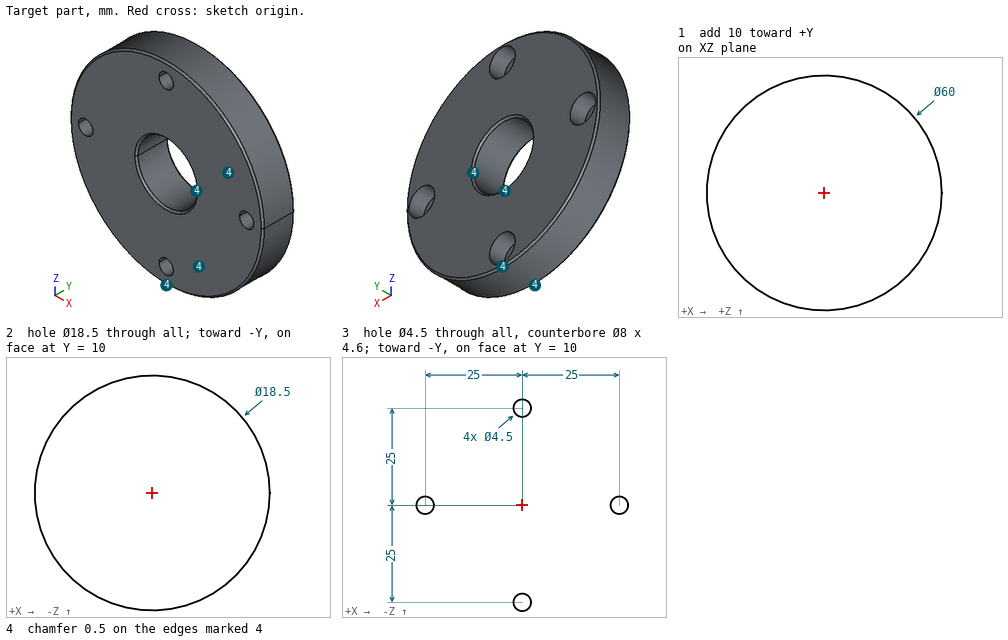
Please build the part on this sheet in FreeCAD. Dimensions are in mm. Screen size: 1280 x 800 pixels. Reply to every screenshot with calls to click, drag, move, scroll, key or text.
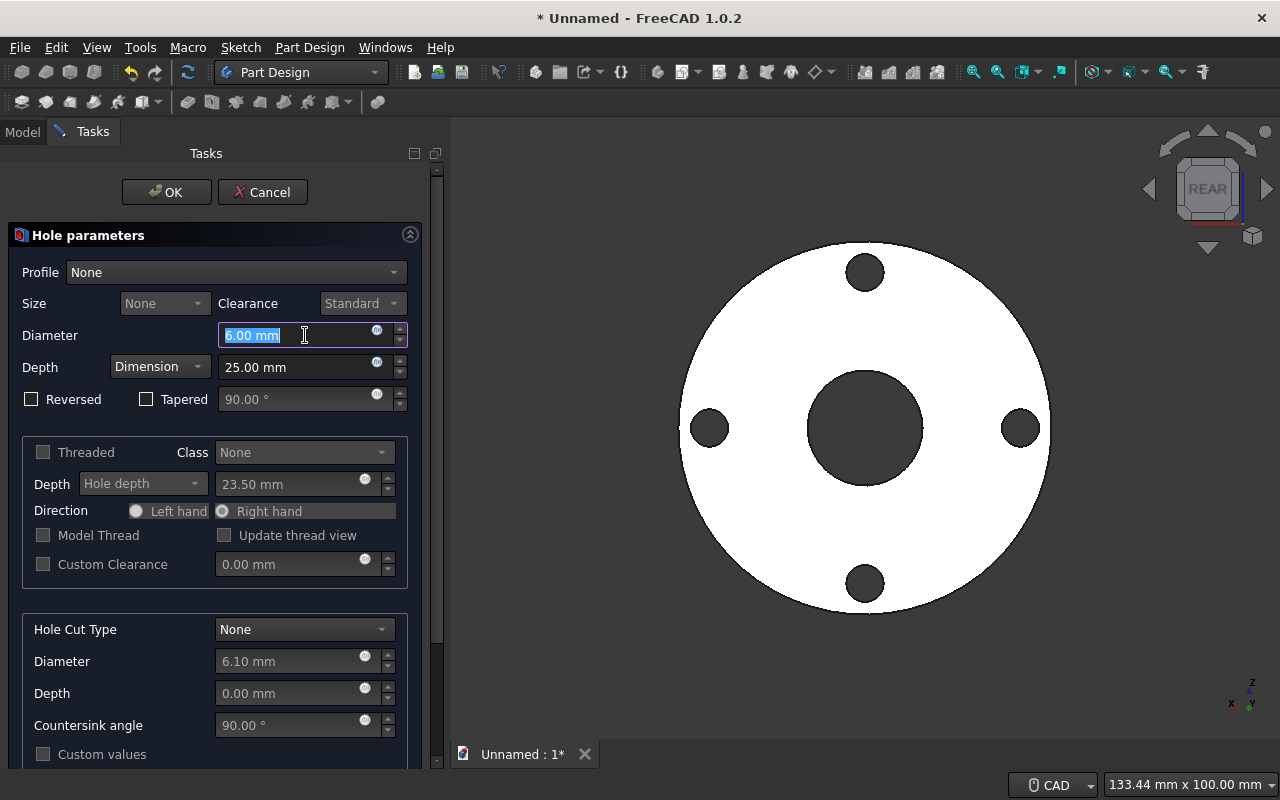
text(4.5)
key(Tab)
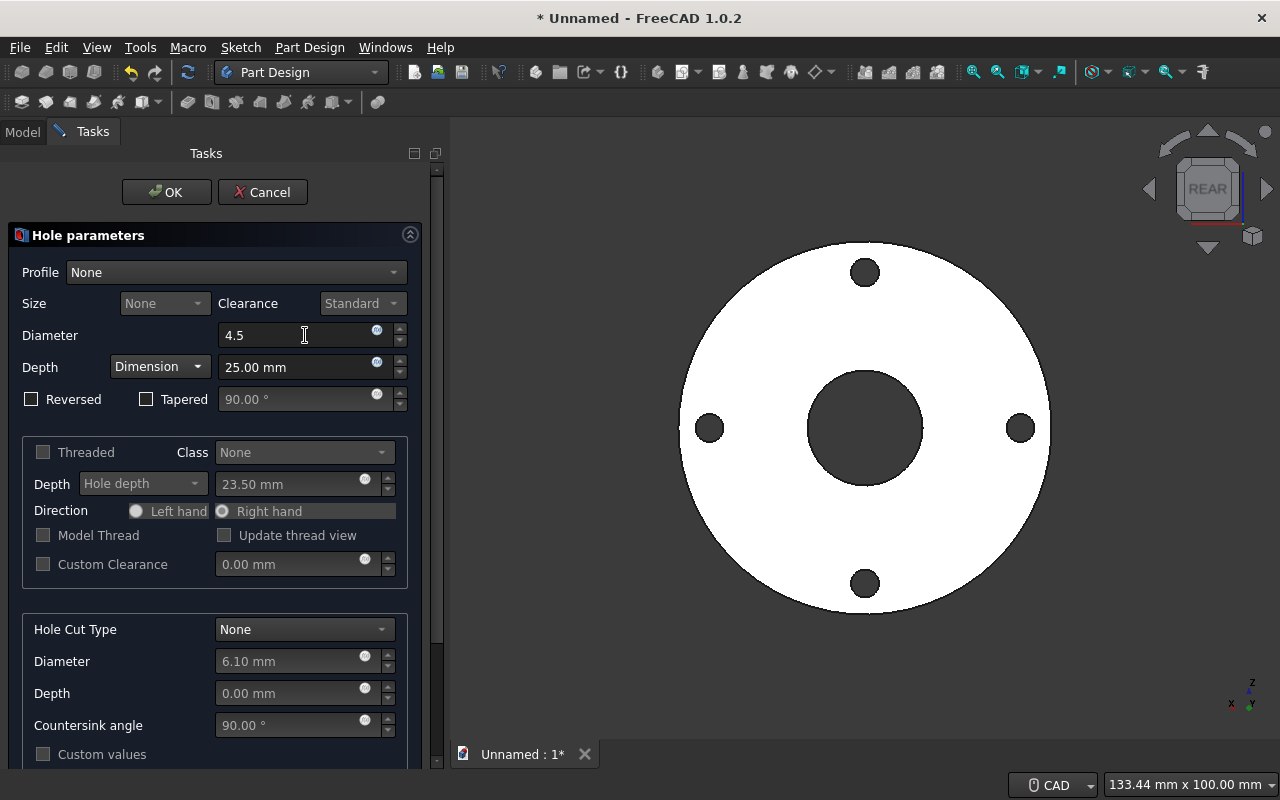
click(161, 366)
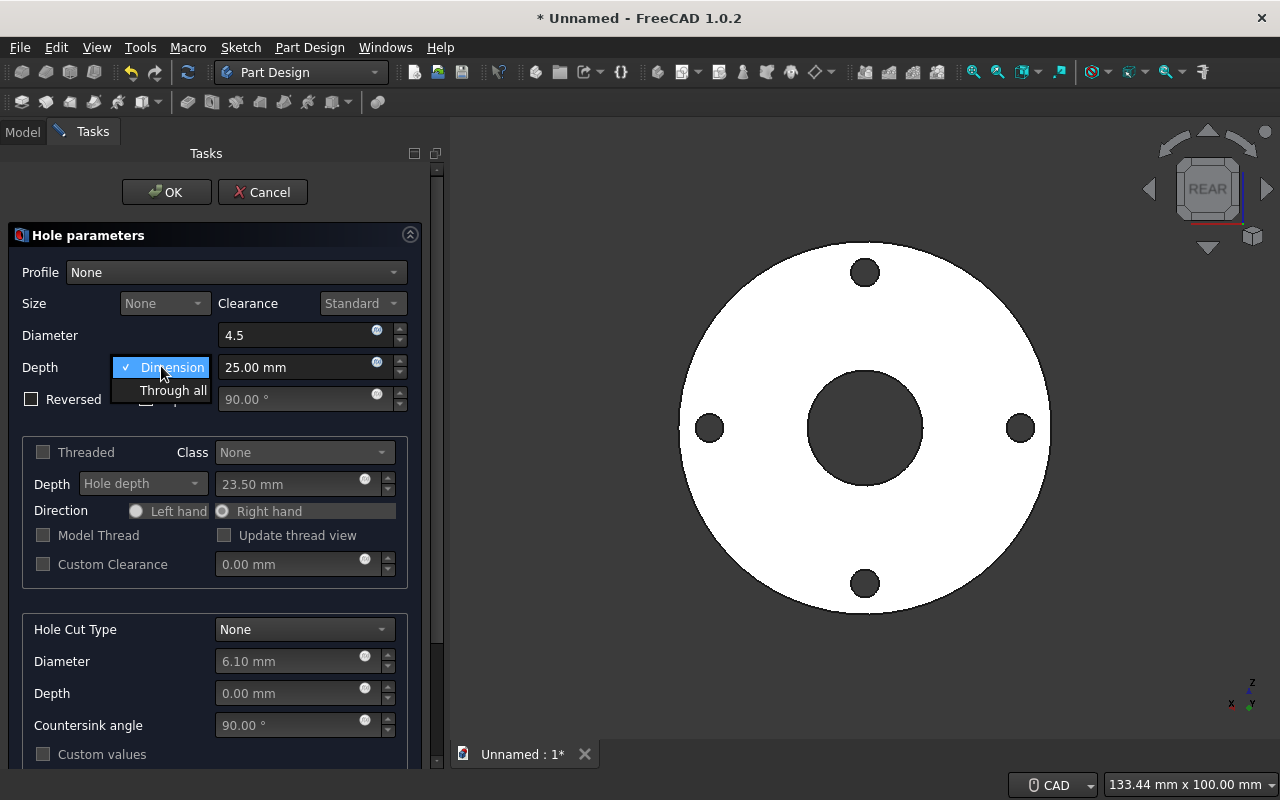
click(160, 390)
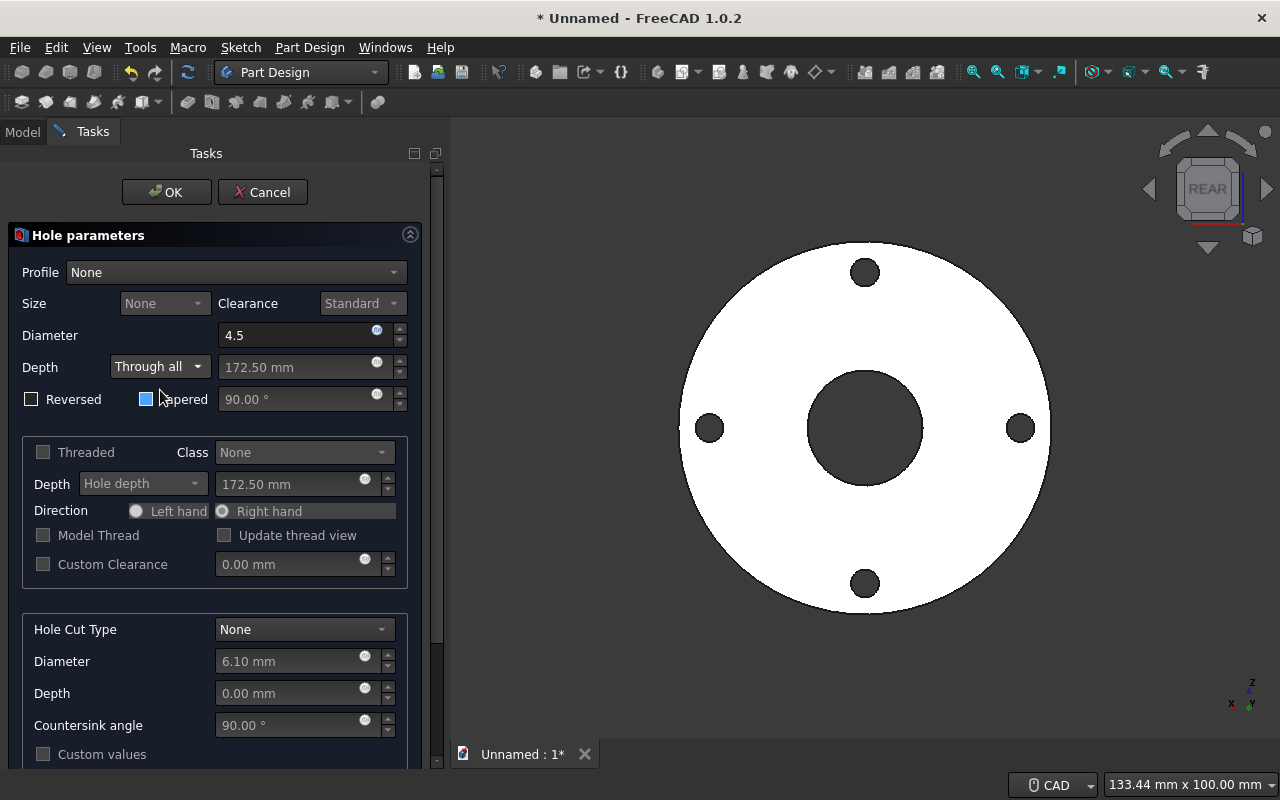
click(306, 630)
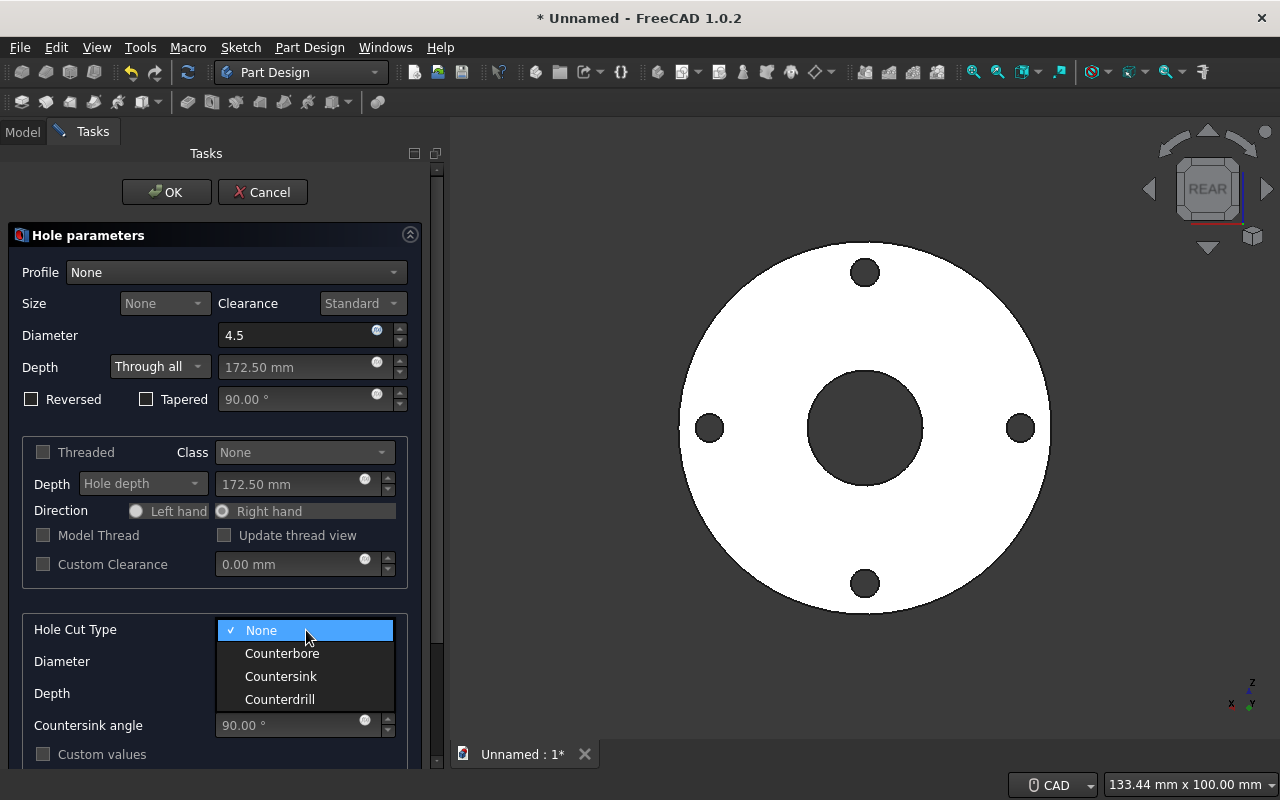
click(304, 654)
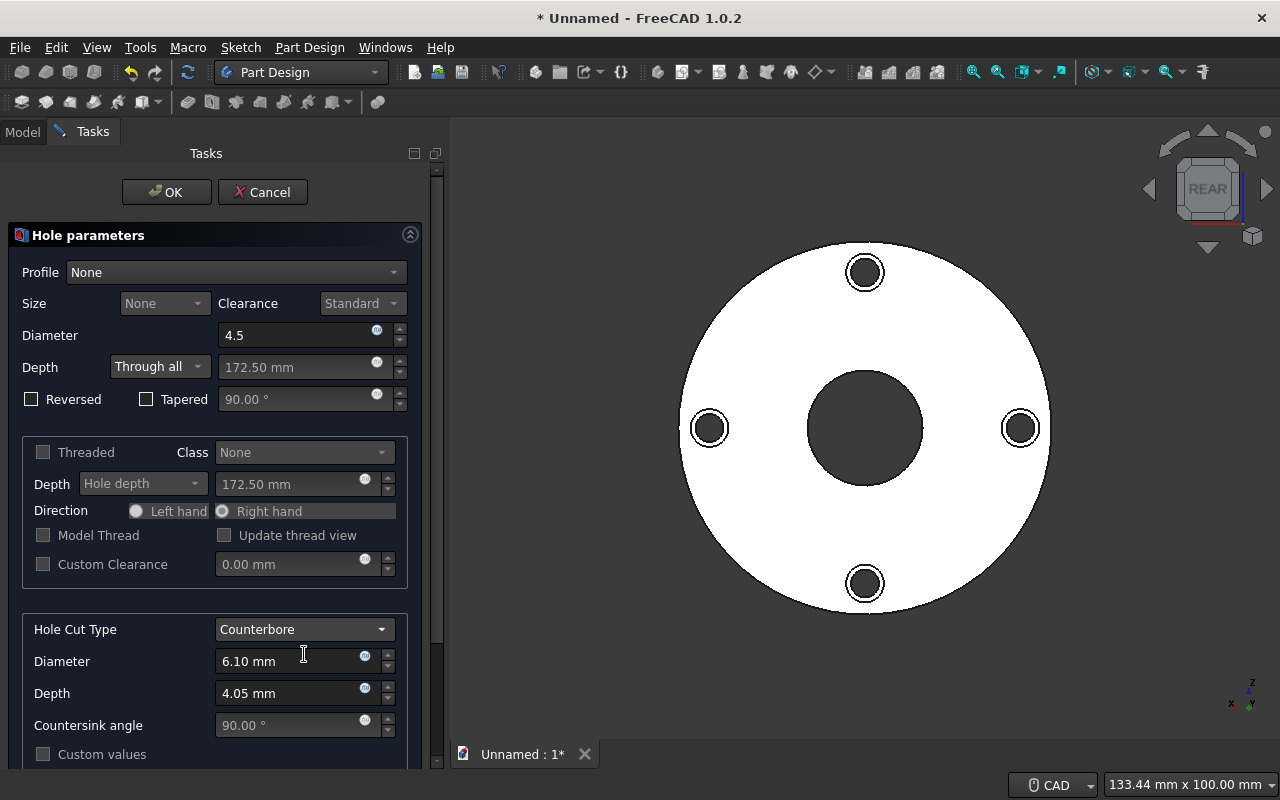
triple_click(298, 661)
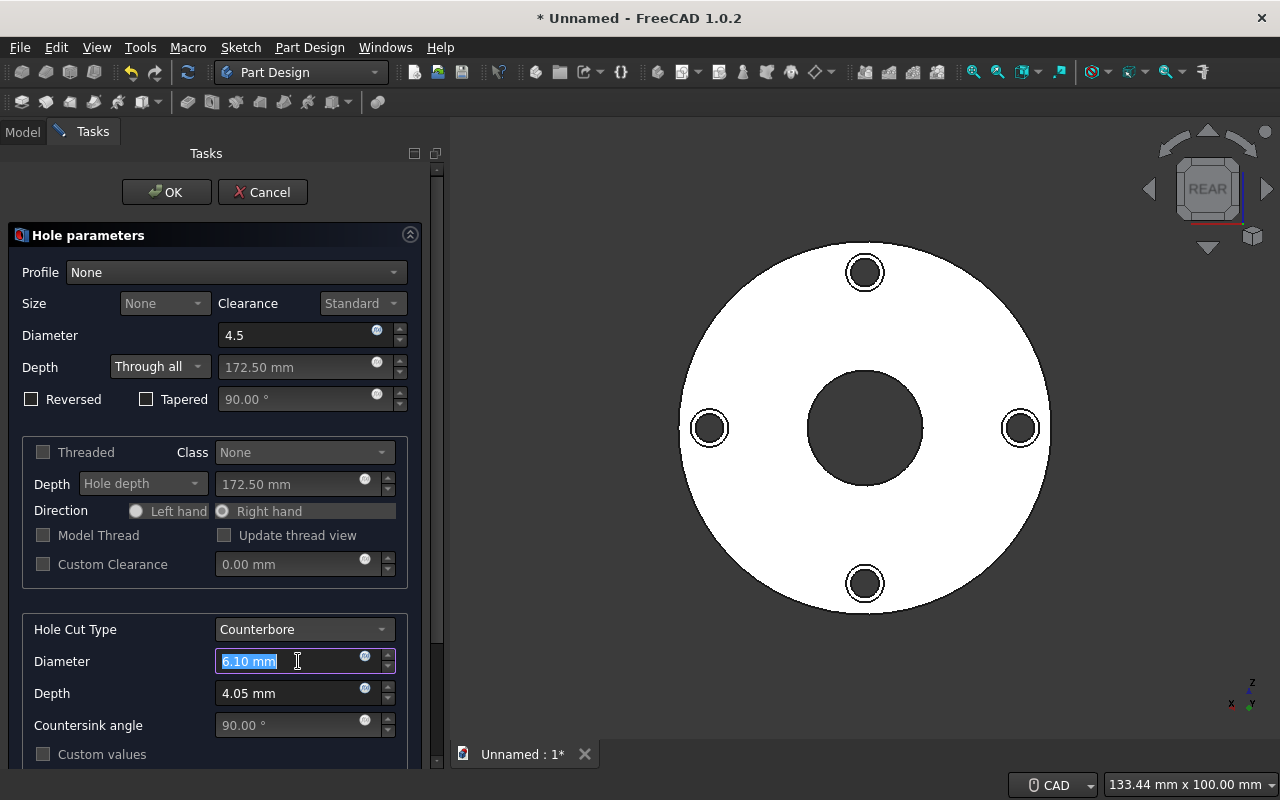
text(8)
key(Tab)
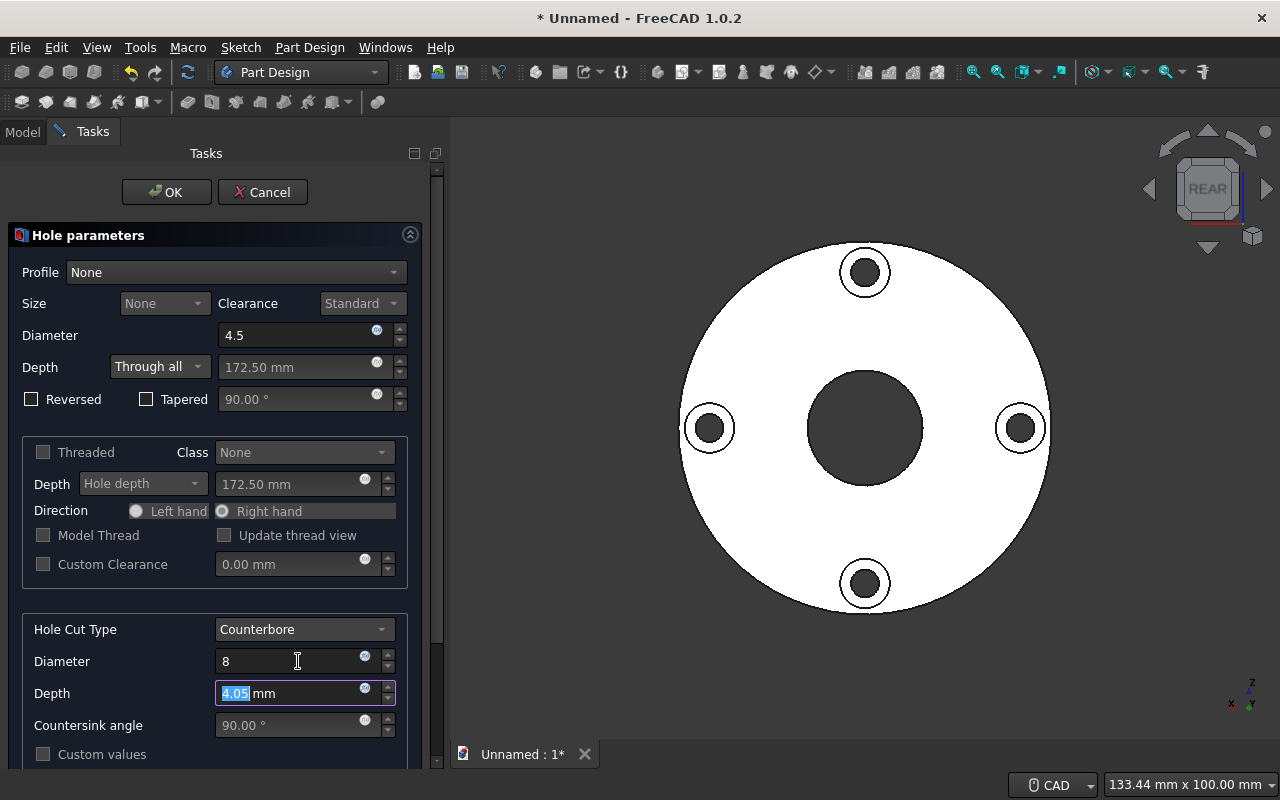
text(4.6)
key(Tab)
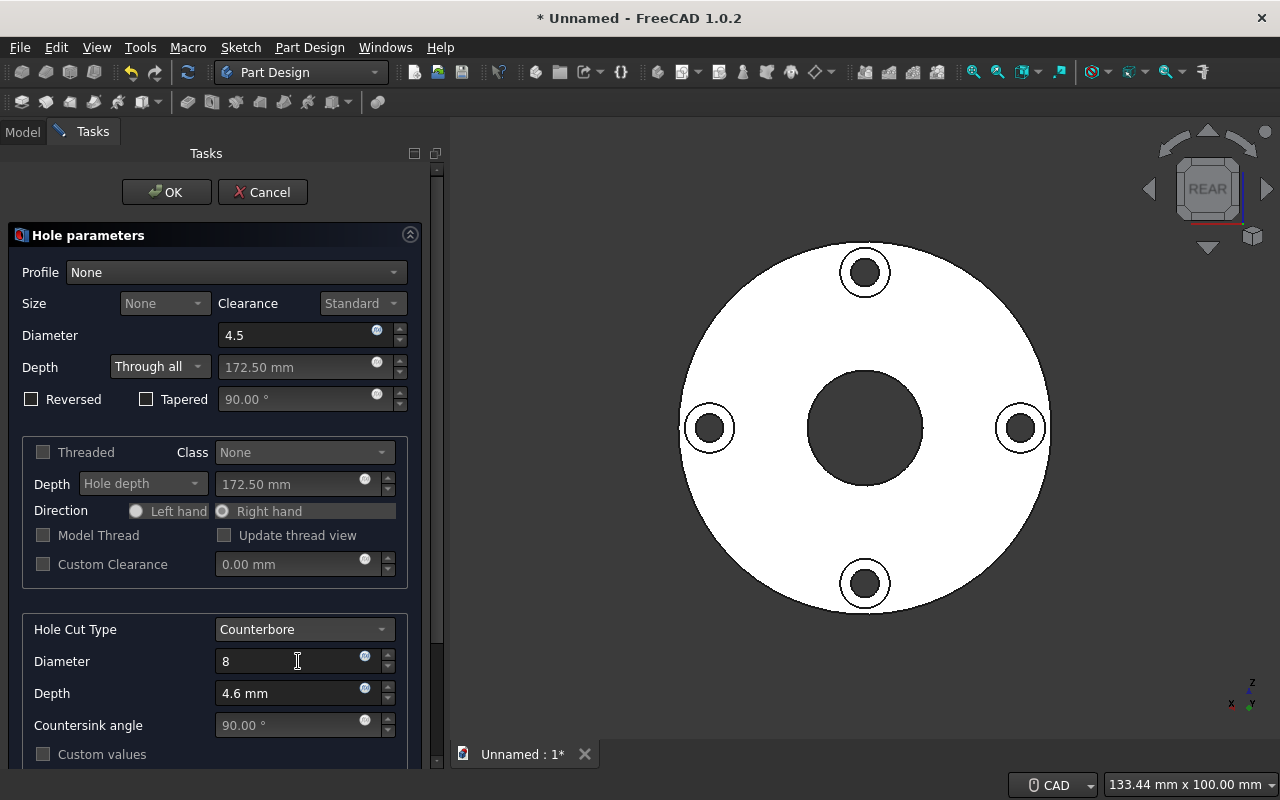
click(167, 192)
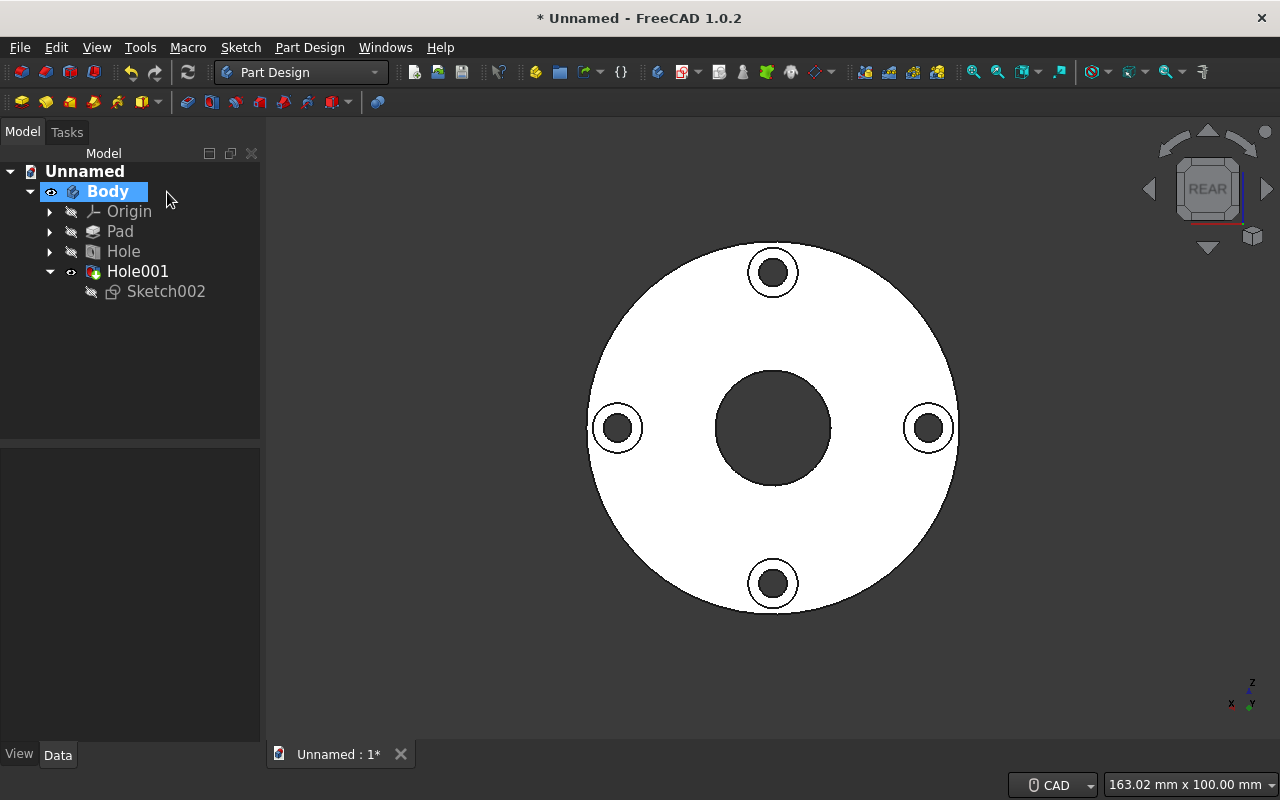
click(960, 427)